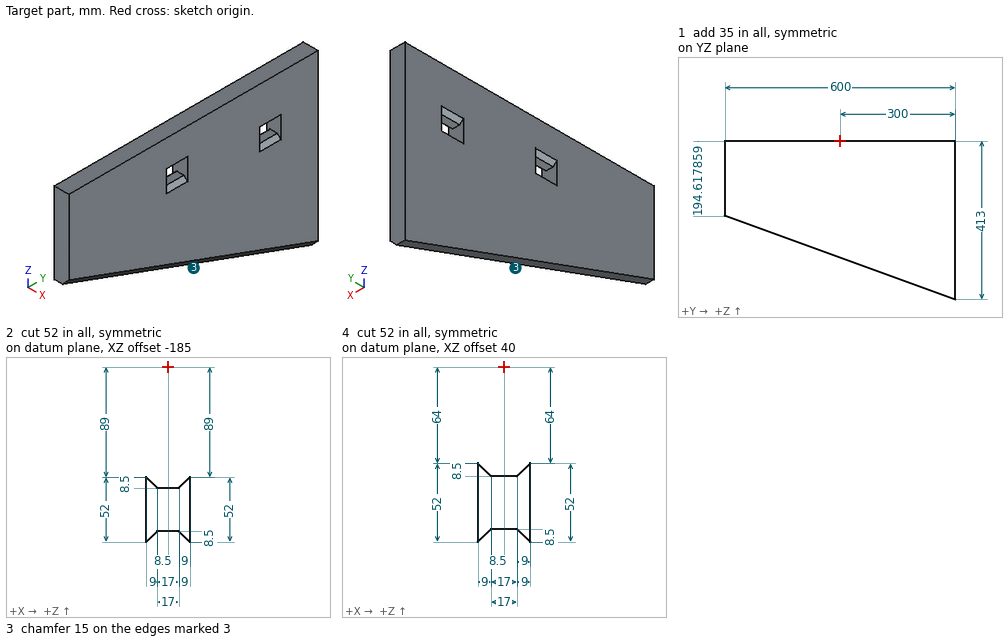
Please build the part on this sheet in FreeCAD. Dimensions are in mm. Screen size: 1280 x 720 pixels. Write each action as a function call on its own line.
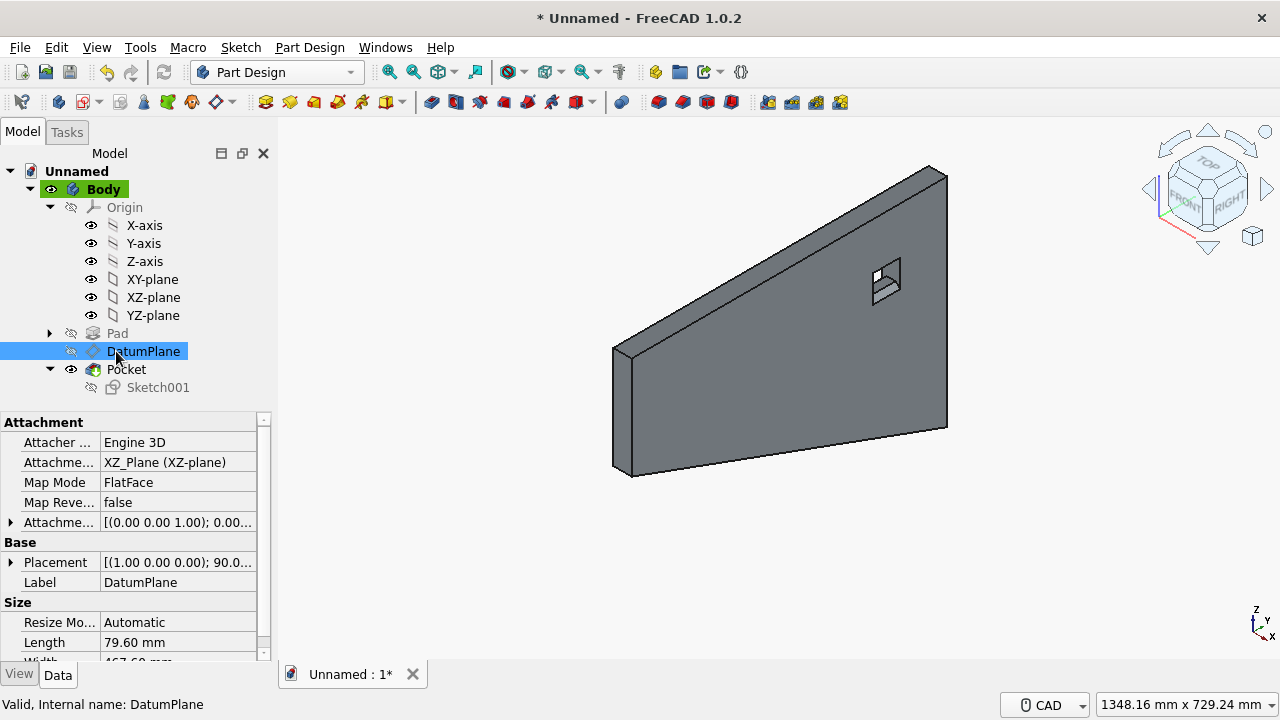
key(2)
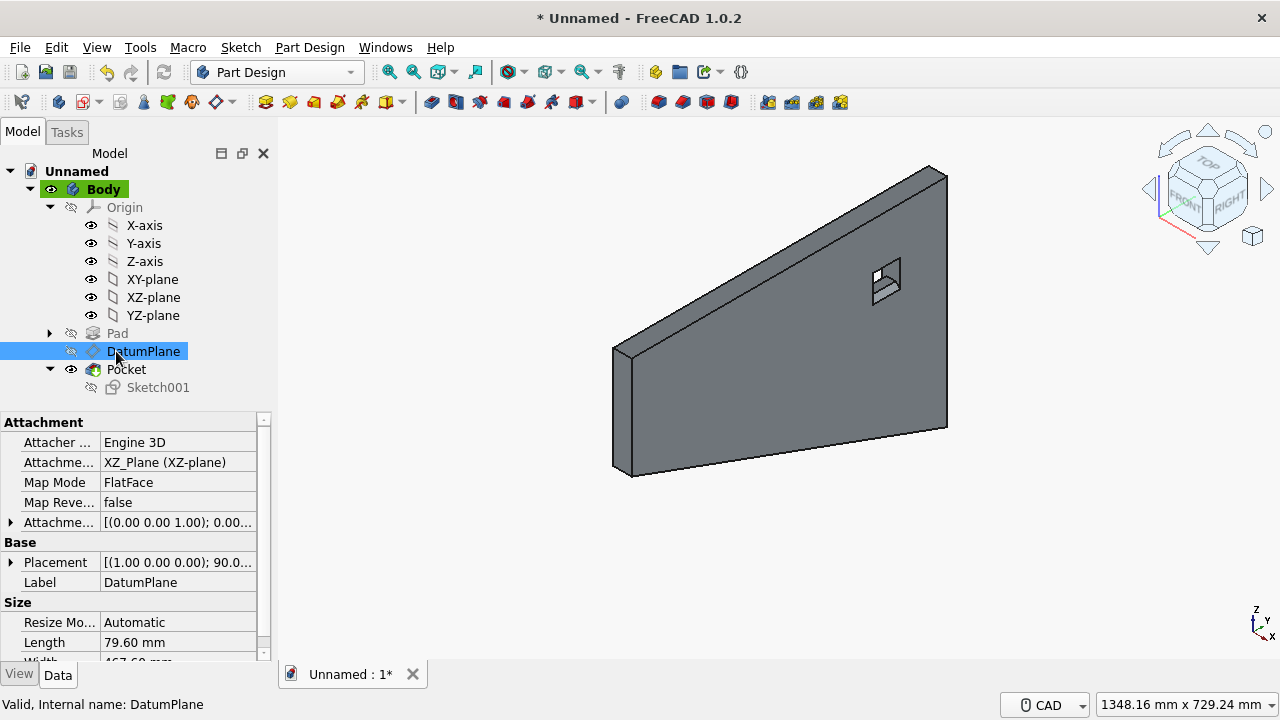
key(1)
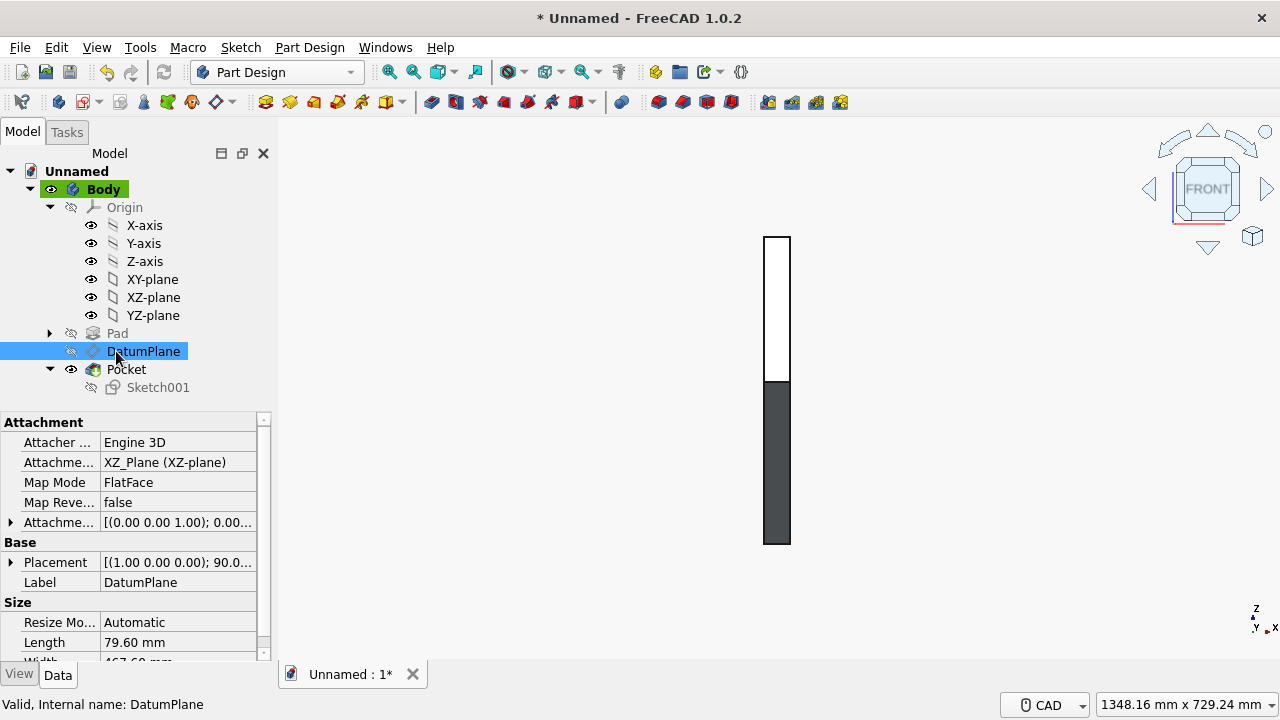
click(790, 462)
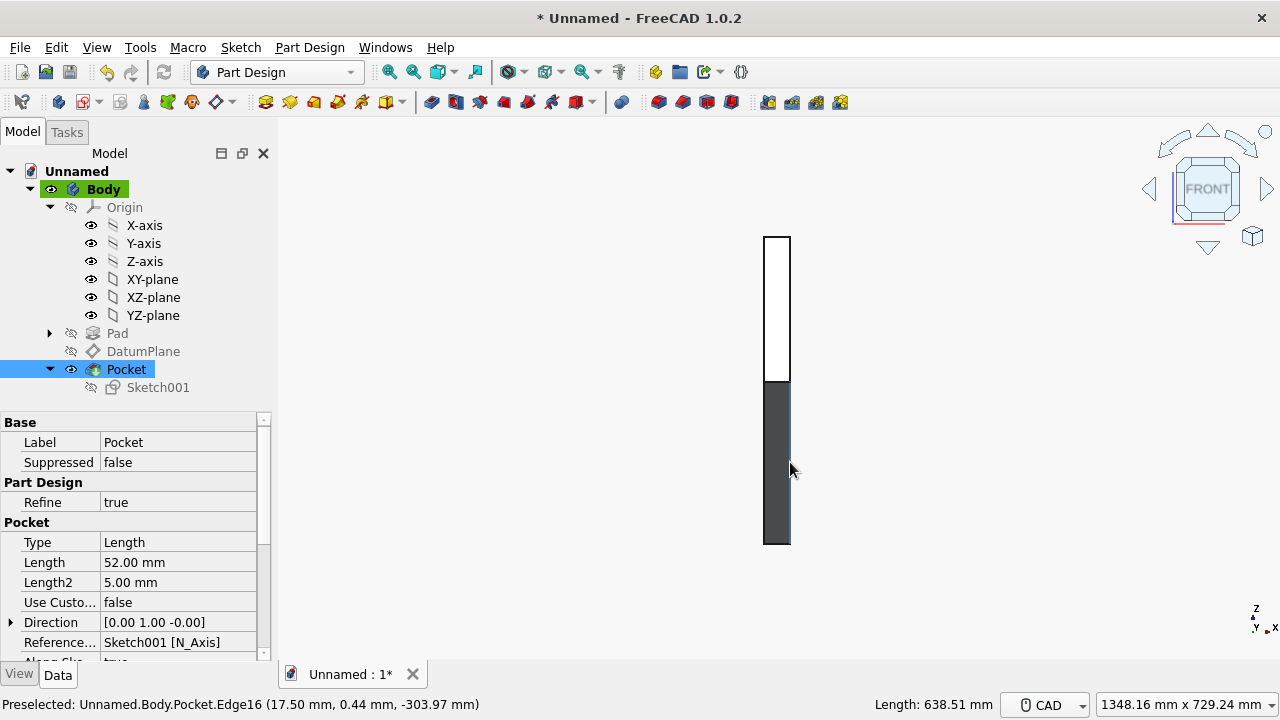
click(684, 102)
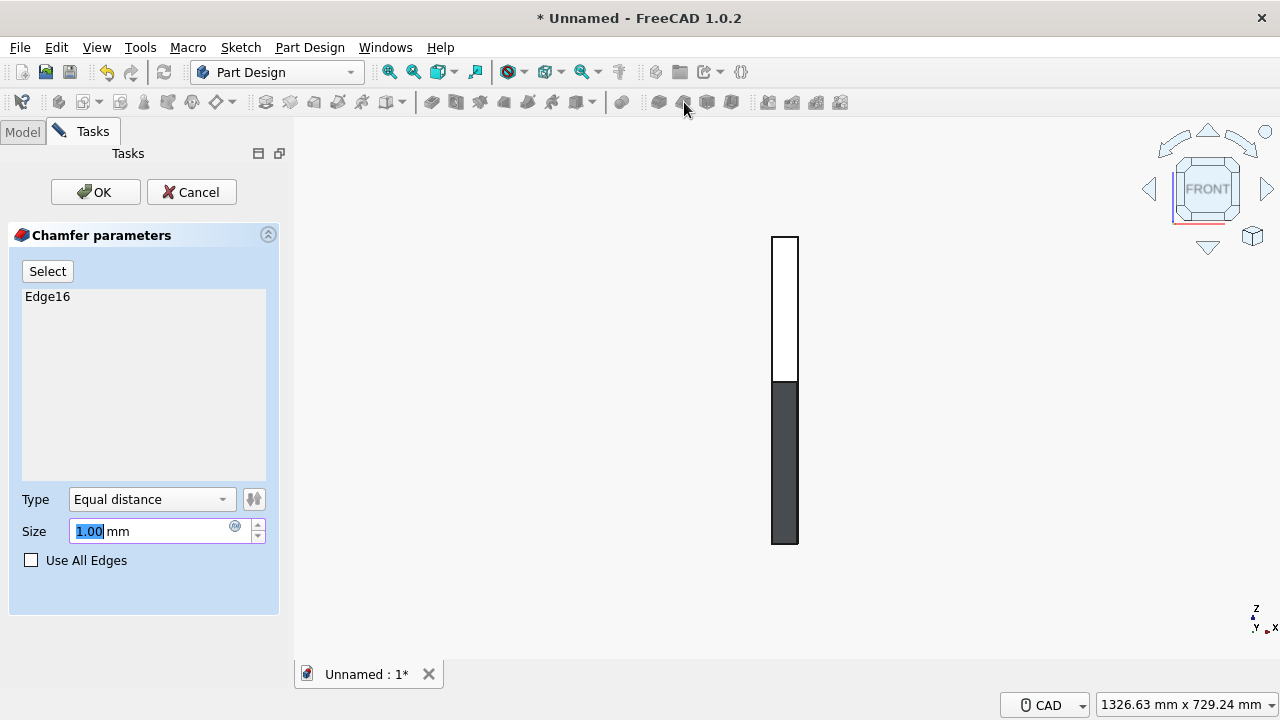
text(15)
key(Tab)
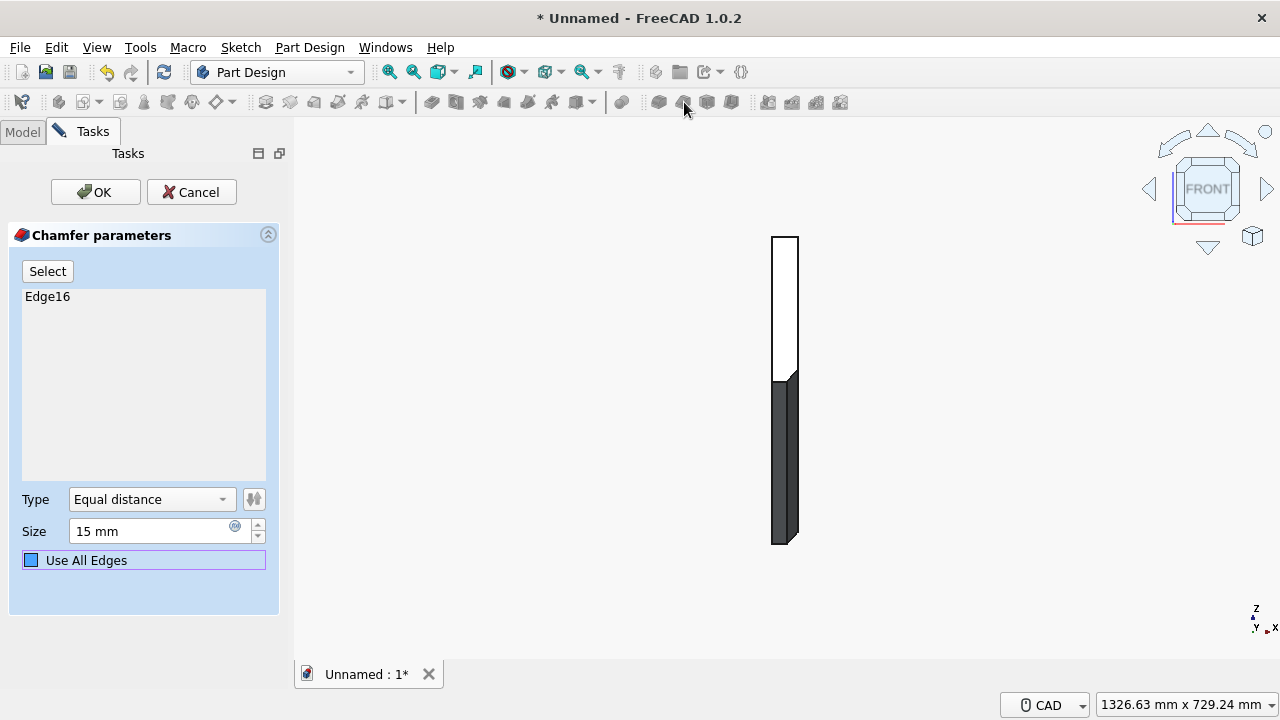
click(96, 192)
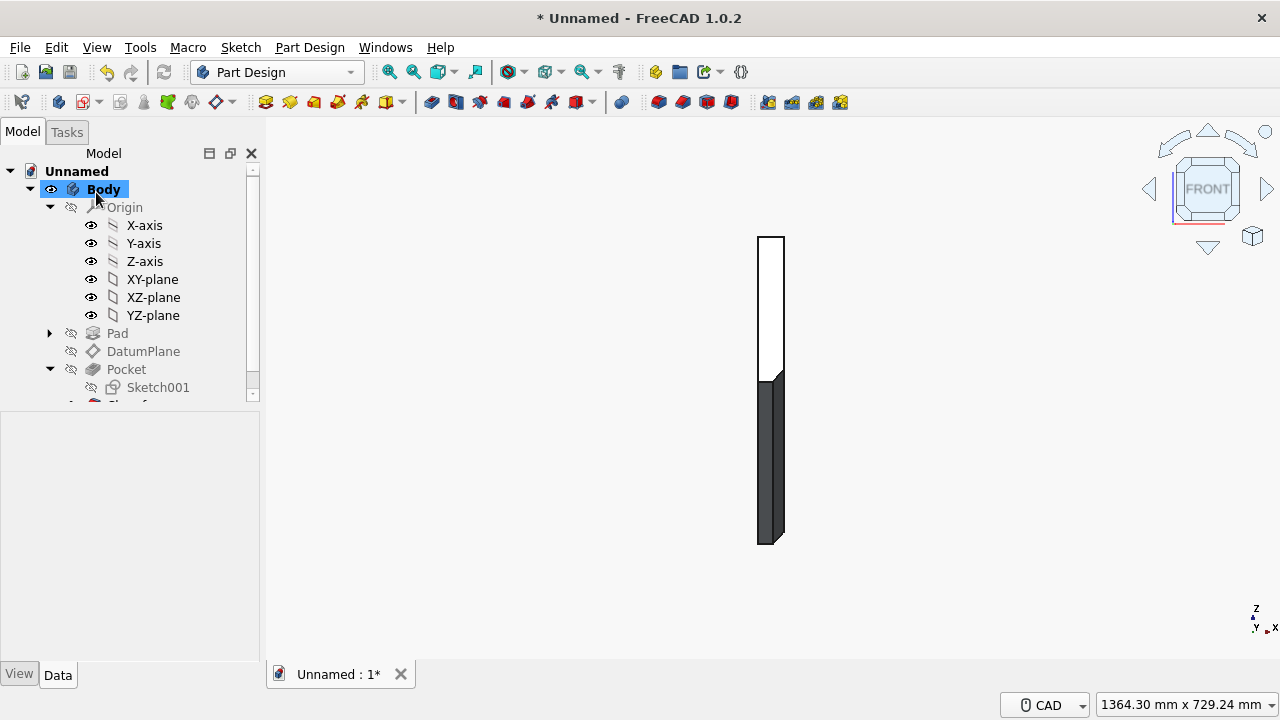
click(136, 297)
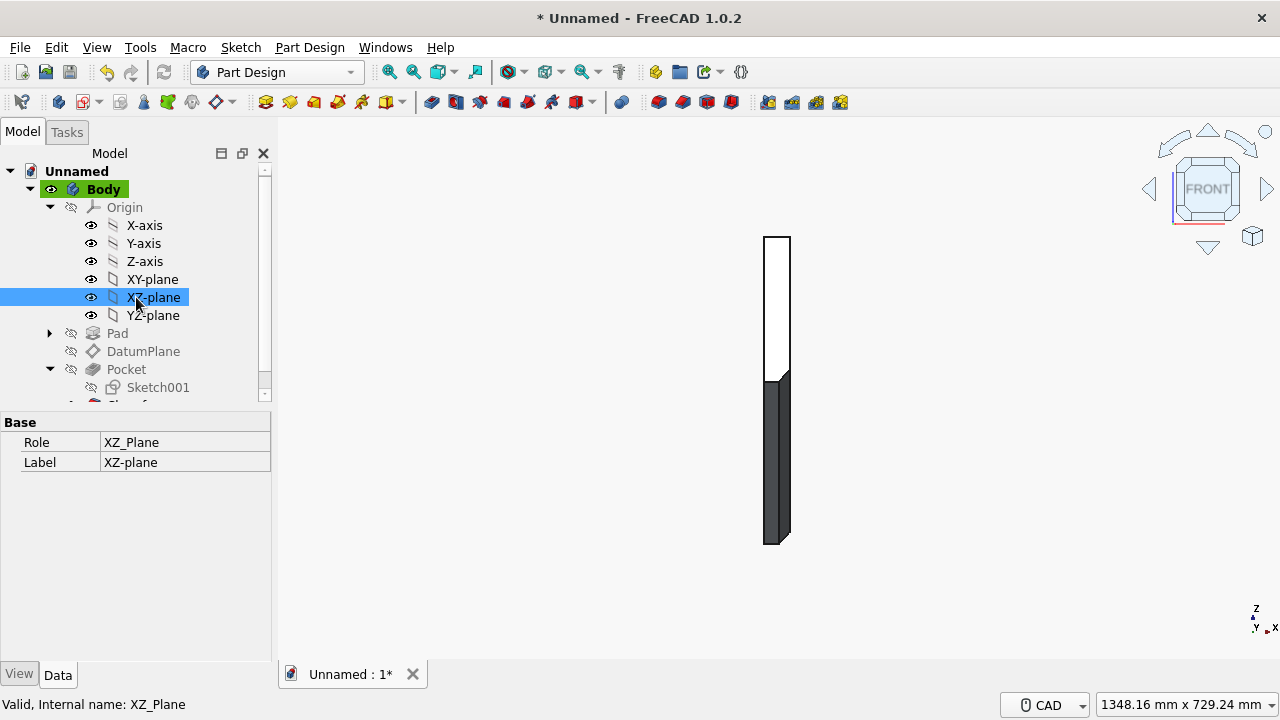
click(216, 102)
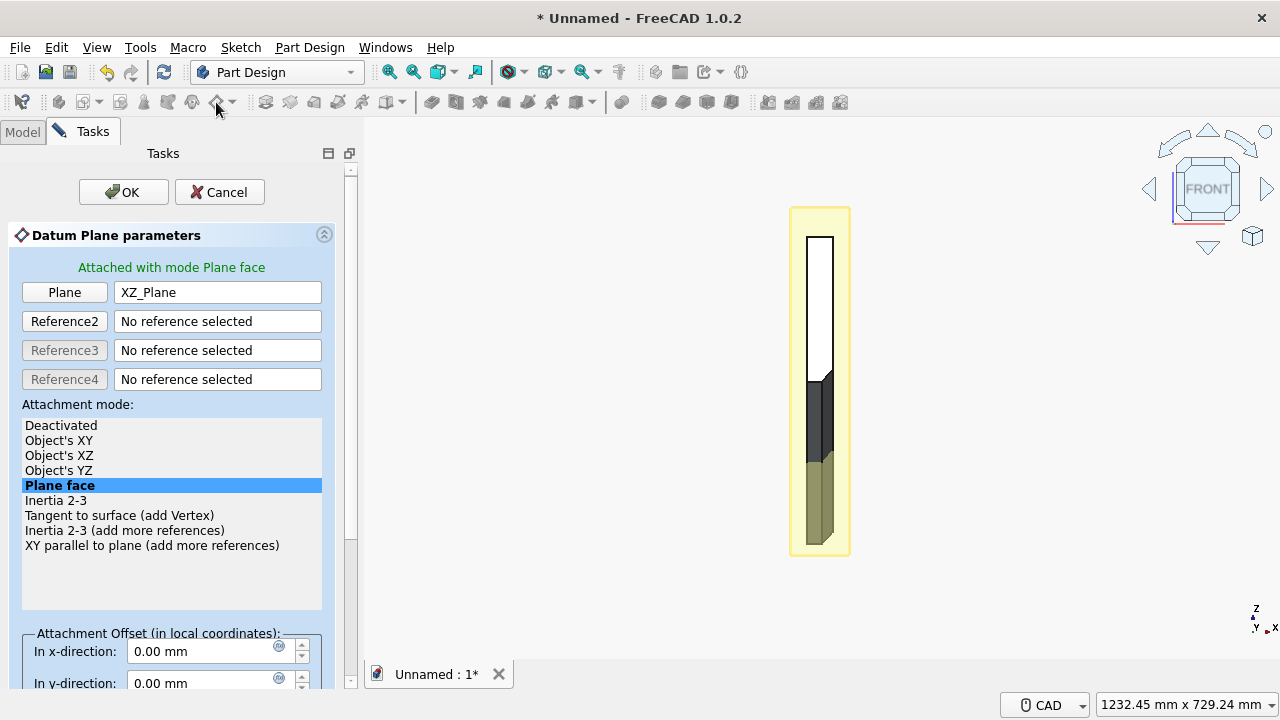
scroll(351, 426, down, 2)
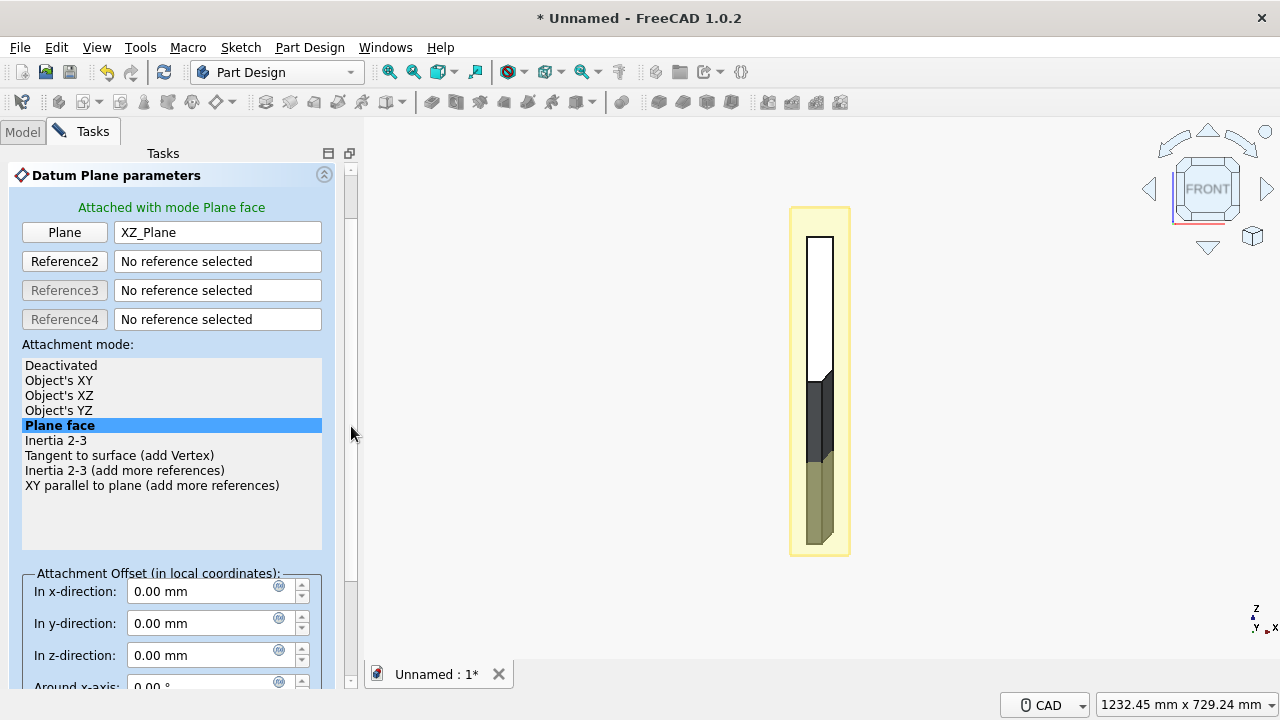
triple_click(210, 595)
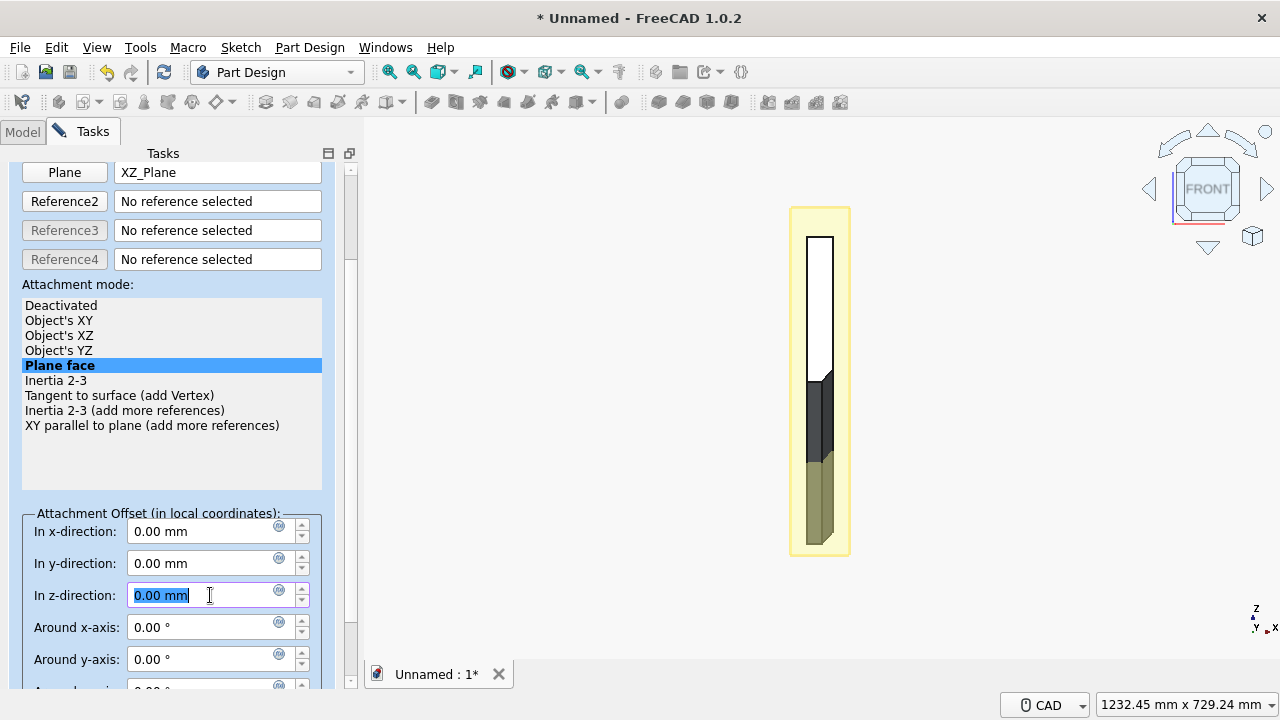
text(40)
key(Tab)